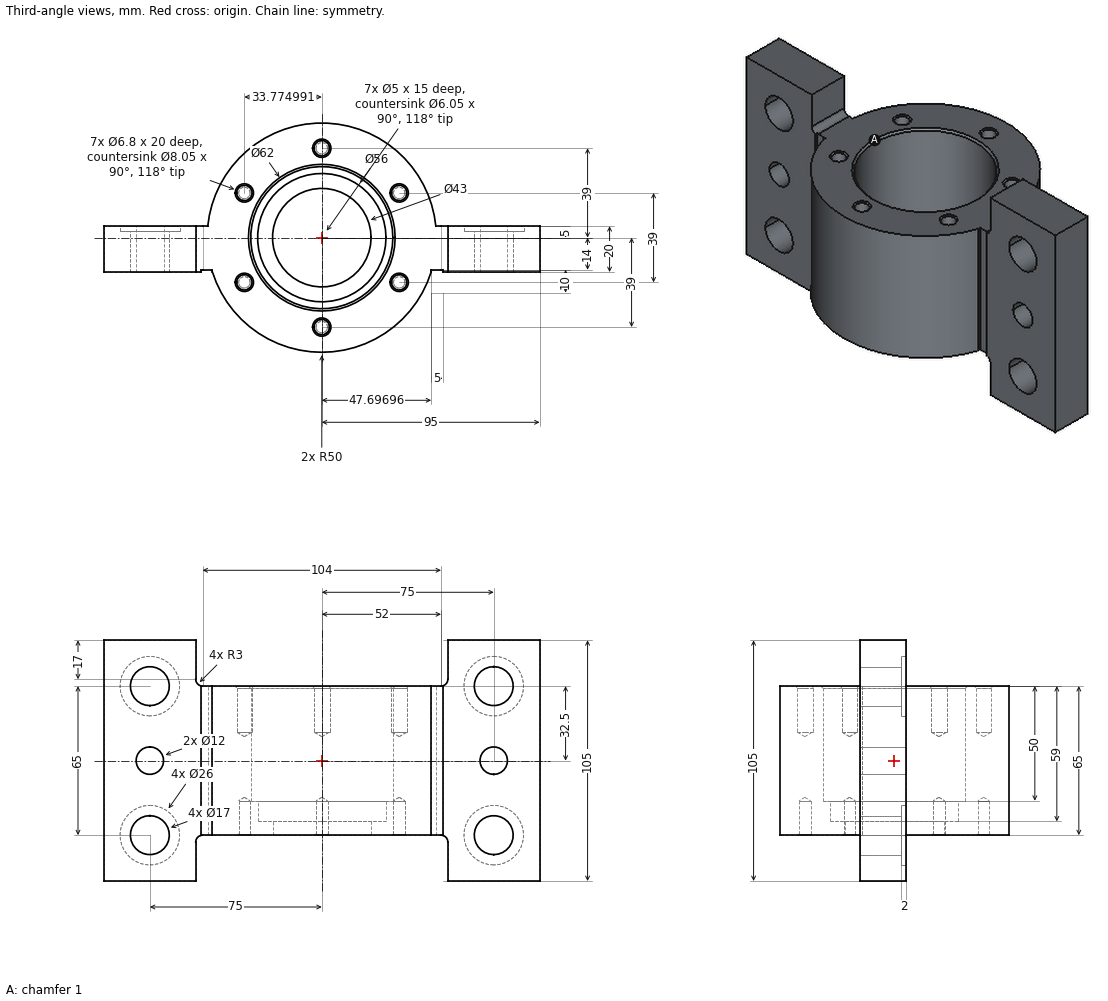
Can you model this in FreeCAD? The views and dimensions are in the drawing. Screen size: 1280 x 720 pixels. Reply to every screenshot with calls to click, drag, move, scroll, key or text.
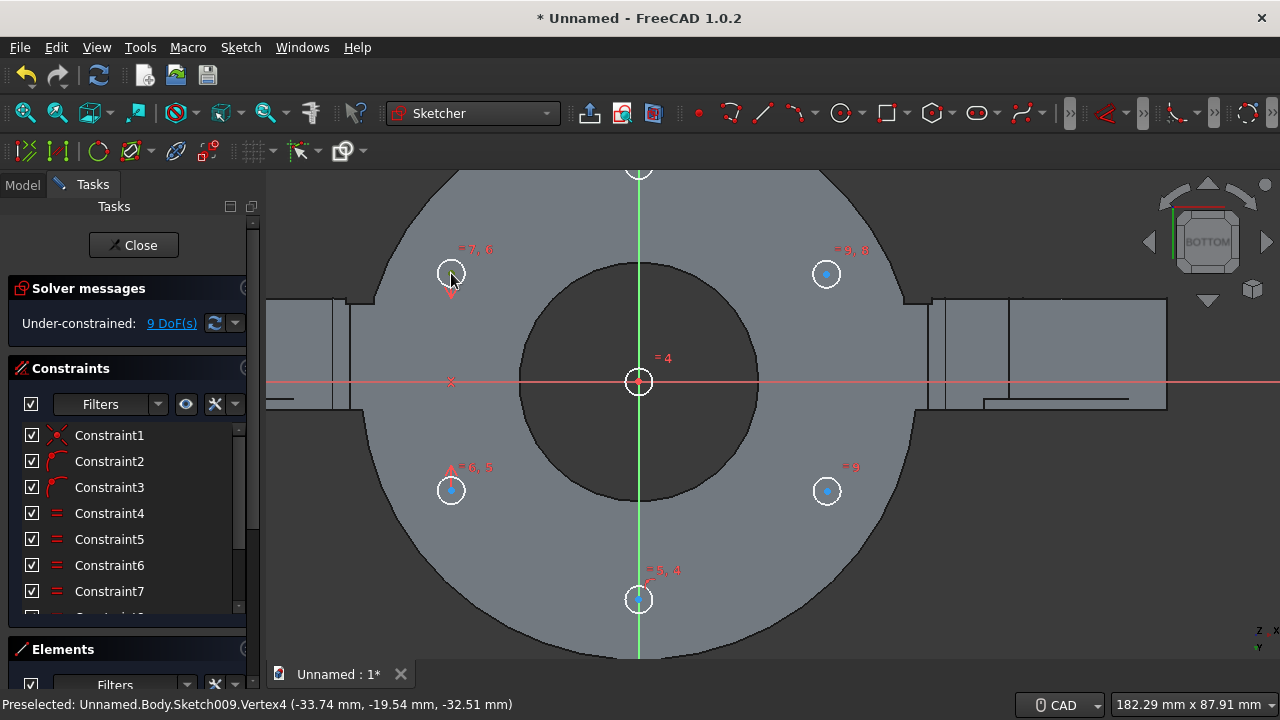
click(827, 274)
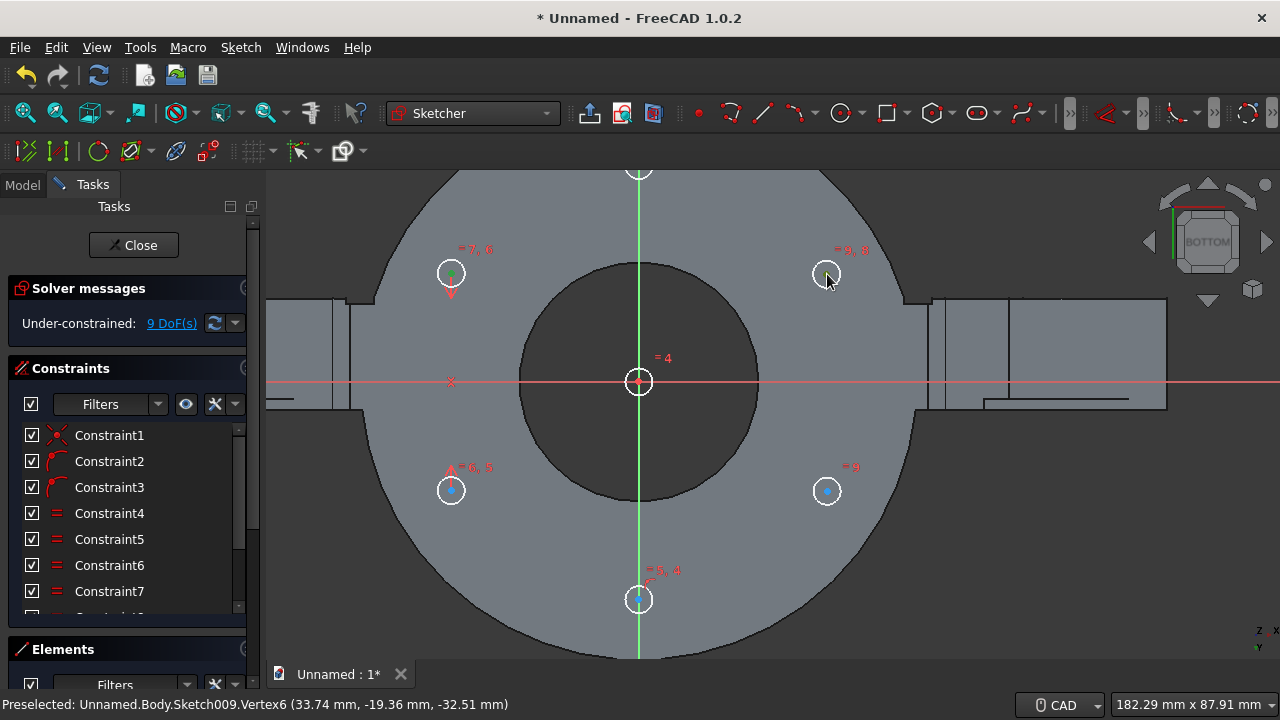
click(639, 538)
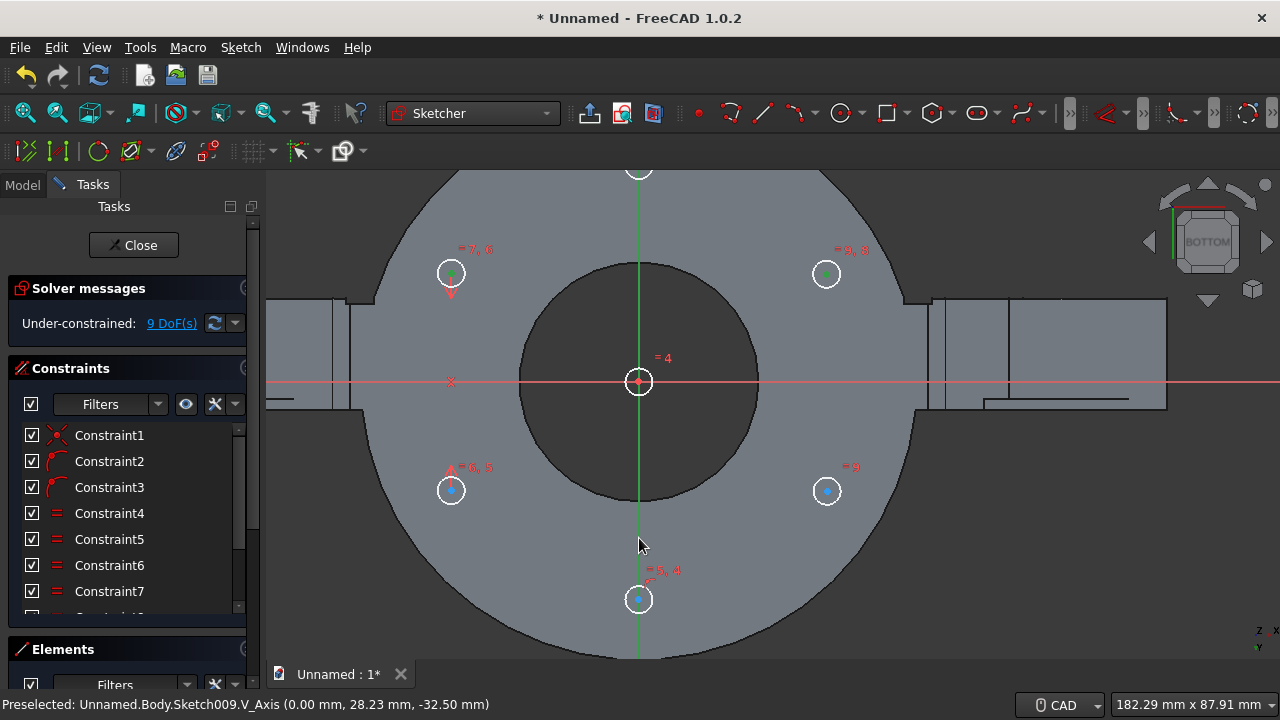
key(s)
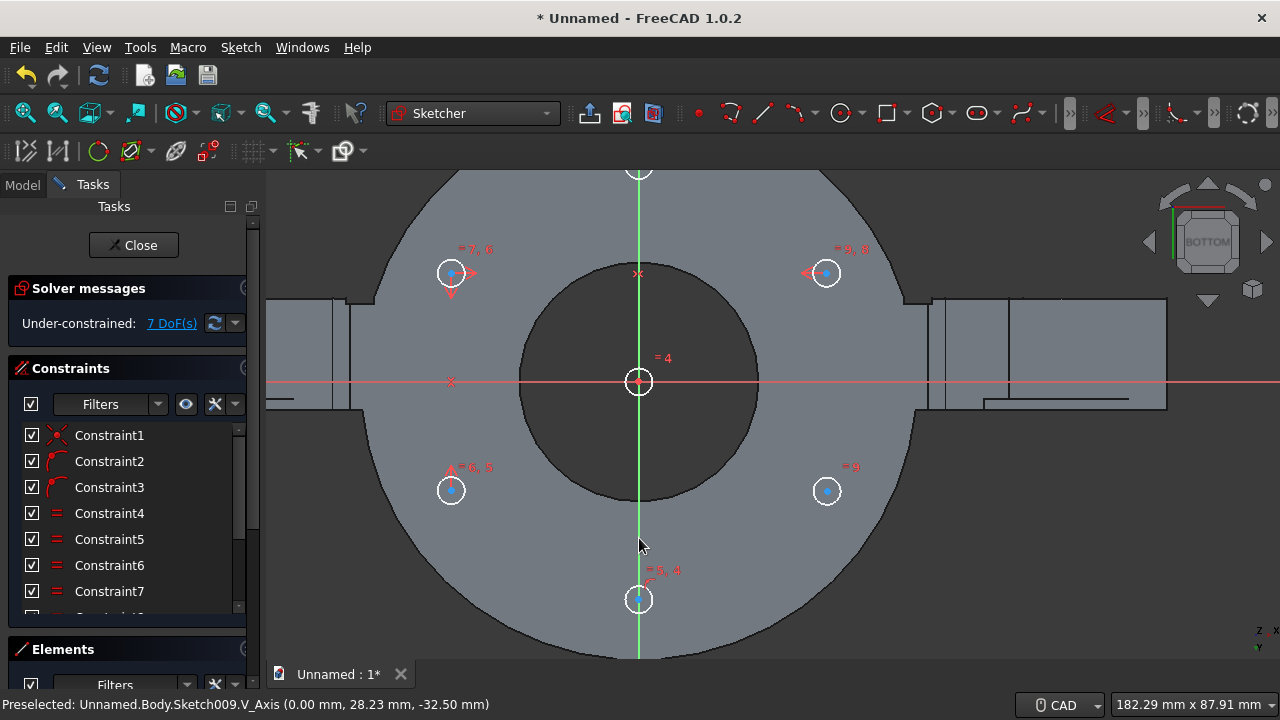
click(451, 491)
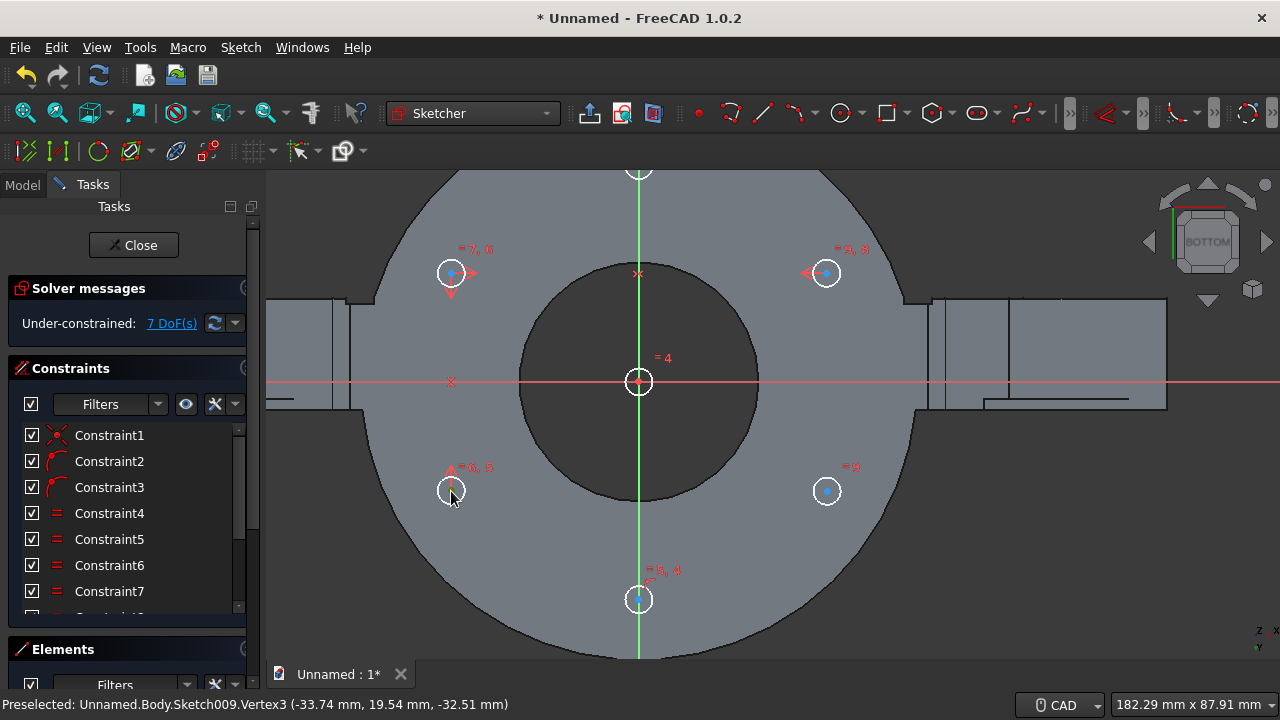
click(827, 491)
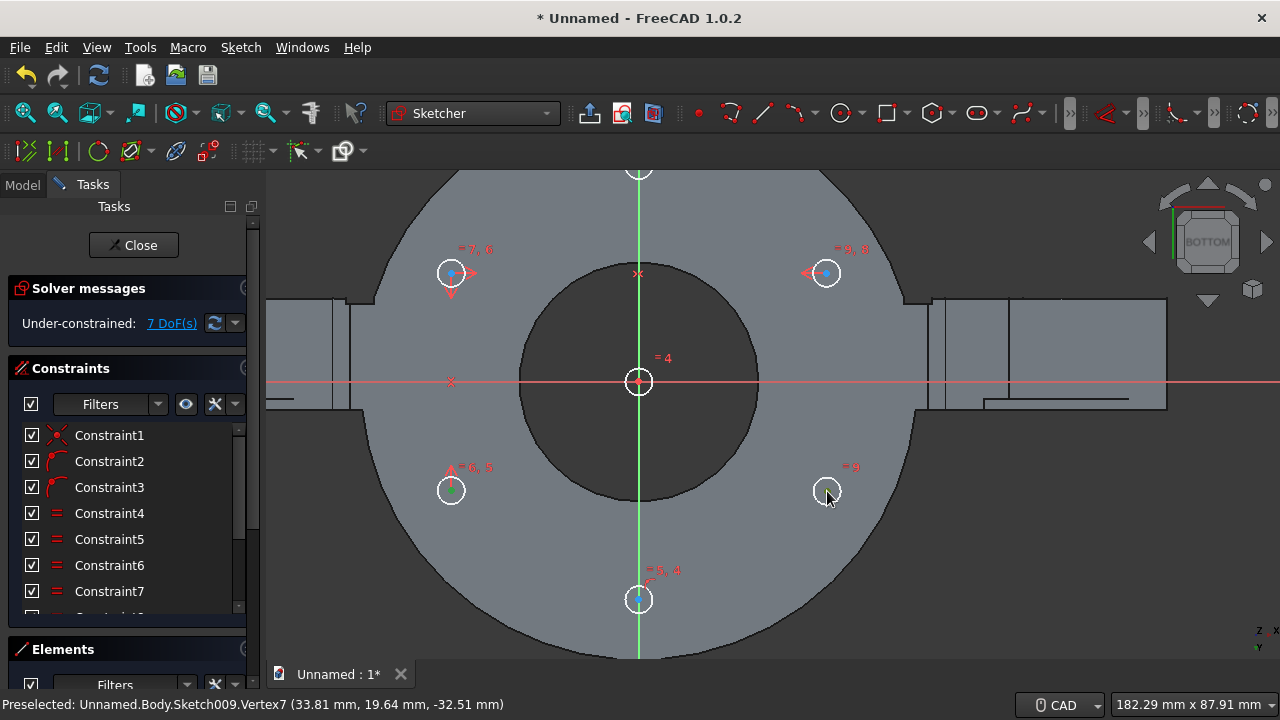
click(639, 538)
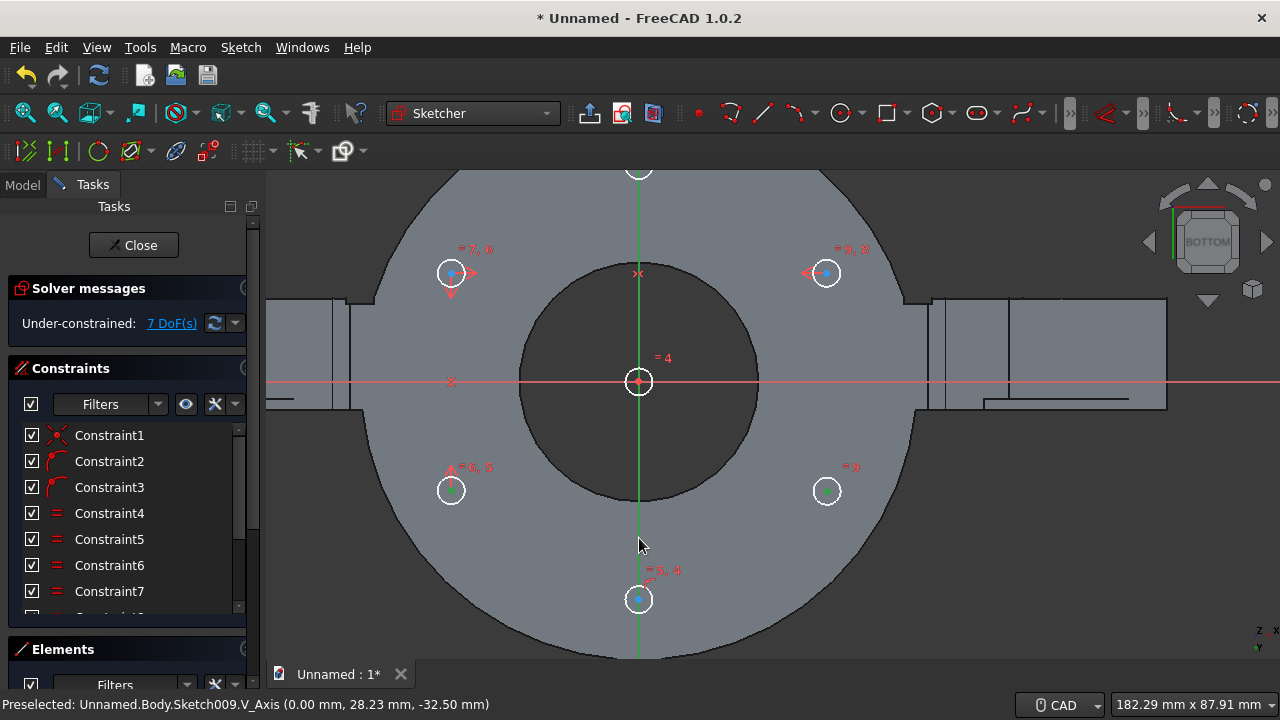
key(s)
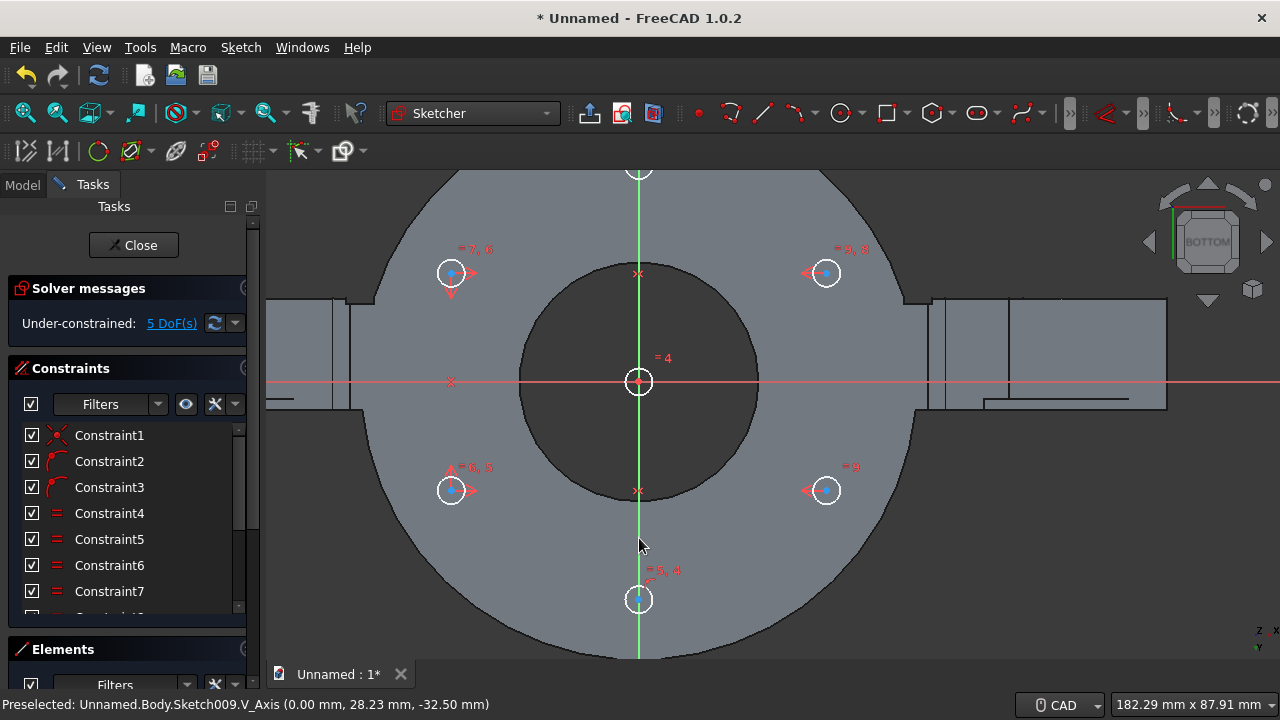
click(1106, 114)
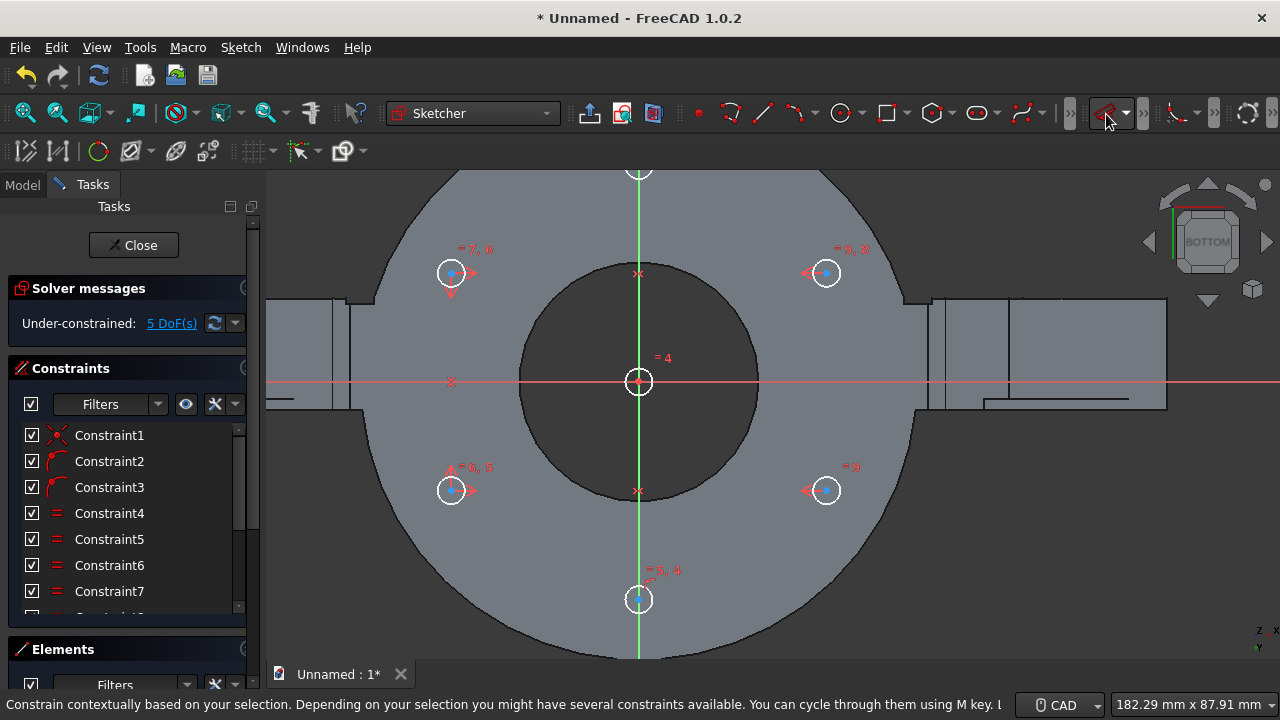
scroll(649, 372, up, 2)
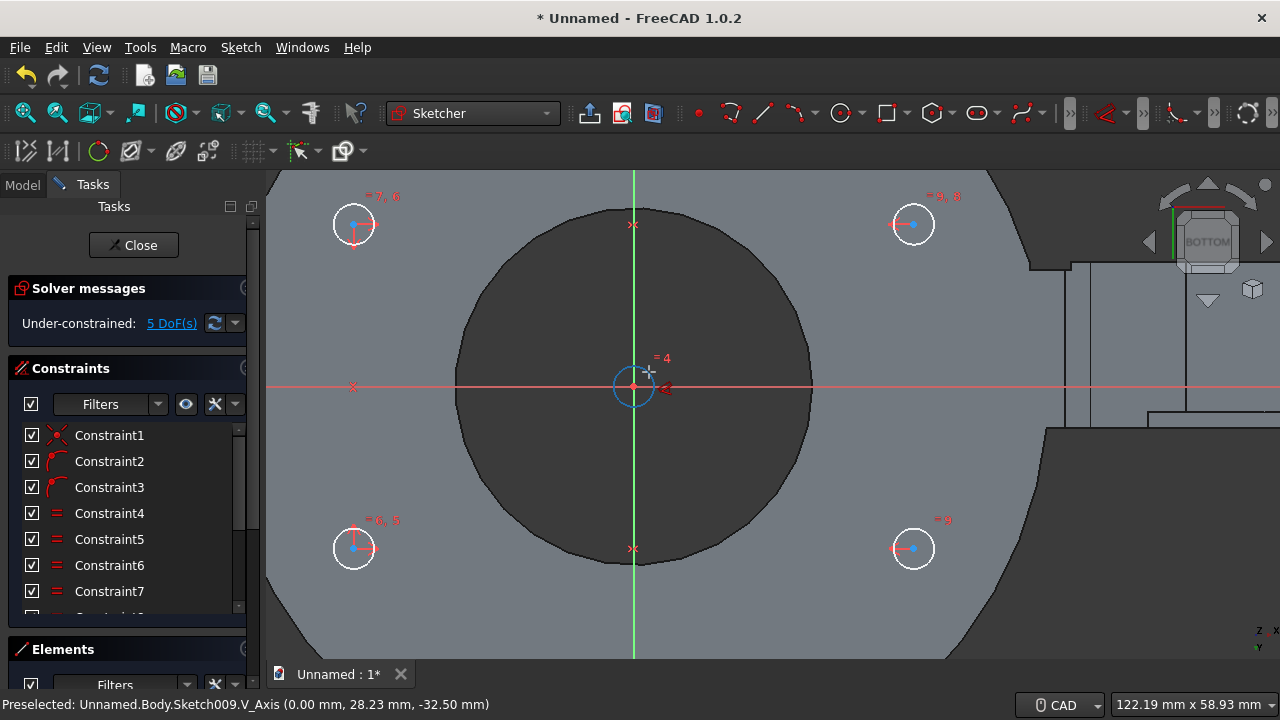
click(648, 372)
click(670, 349)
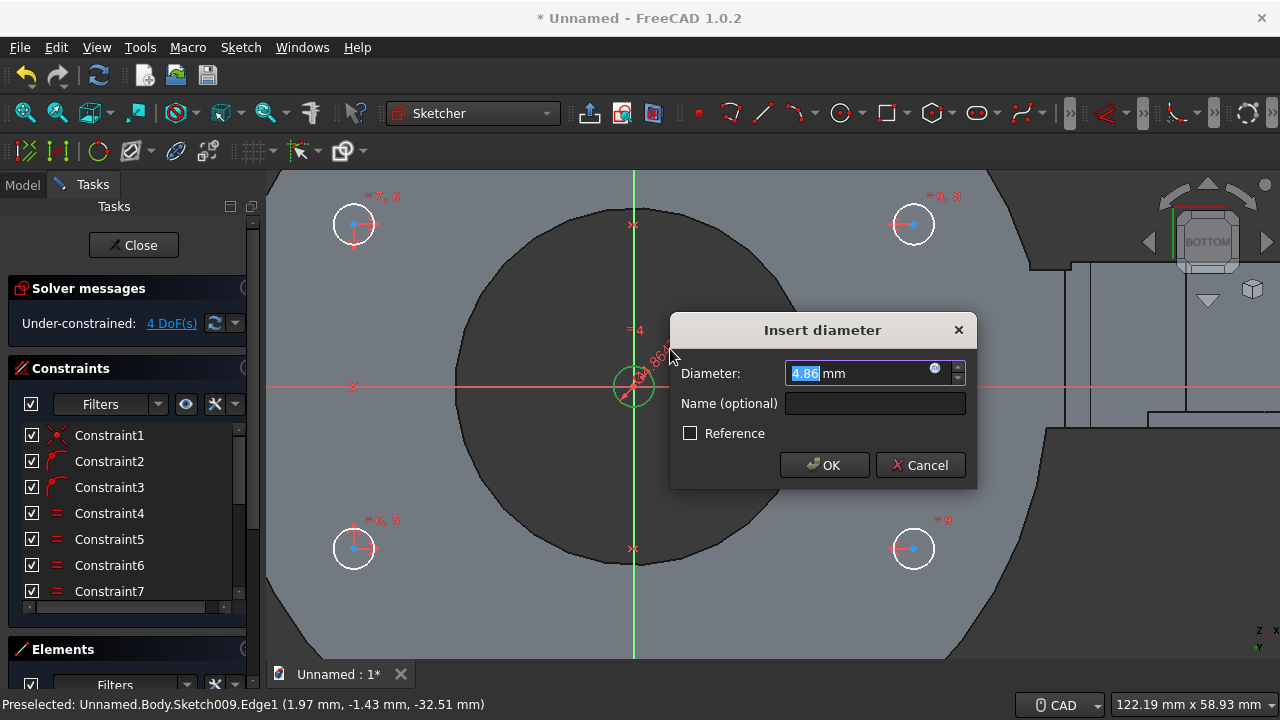
text(5)
key(Return)